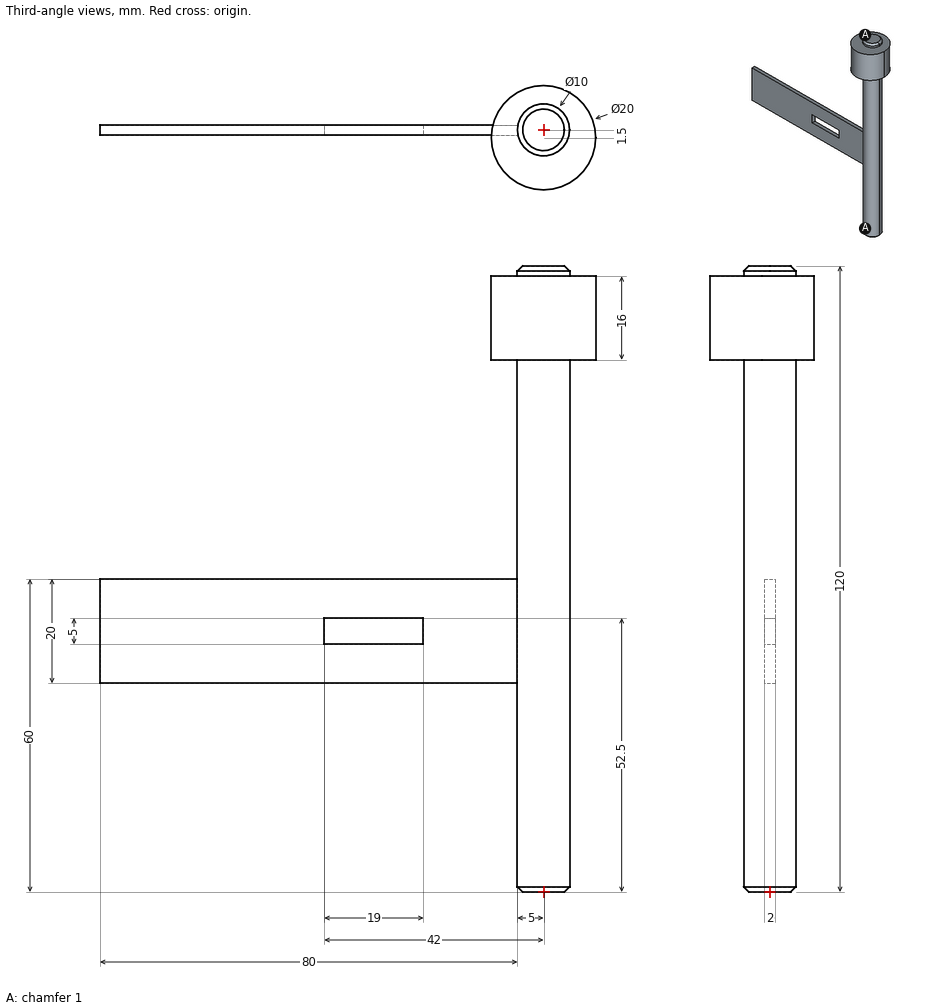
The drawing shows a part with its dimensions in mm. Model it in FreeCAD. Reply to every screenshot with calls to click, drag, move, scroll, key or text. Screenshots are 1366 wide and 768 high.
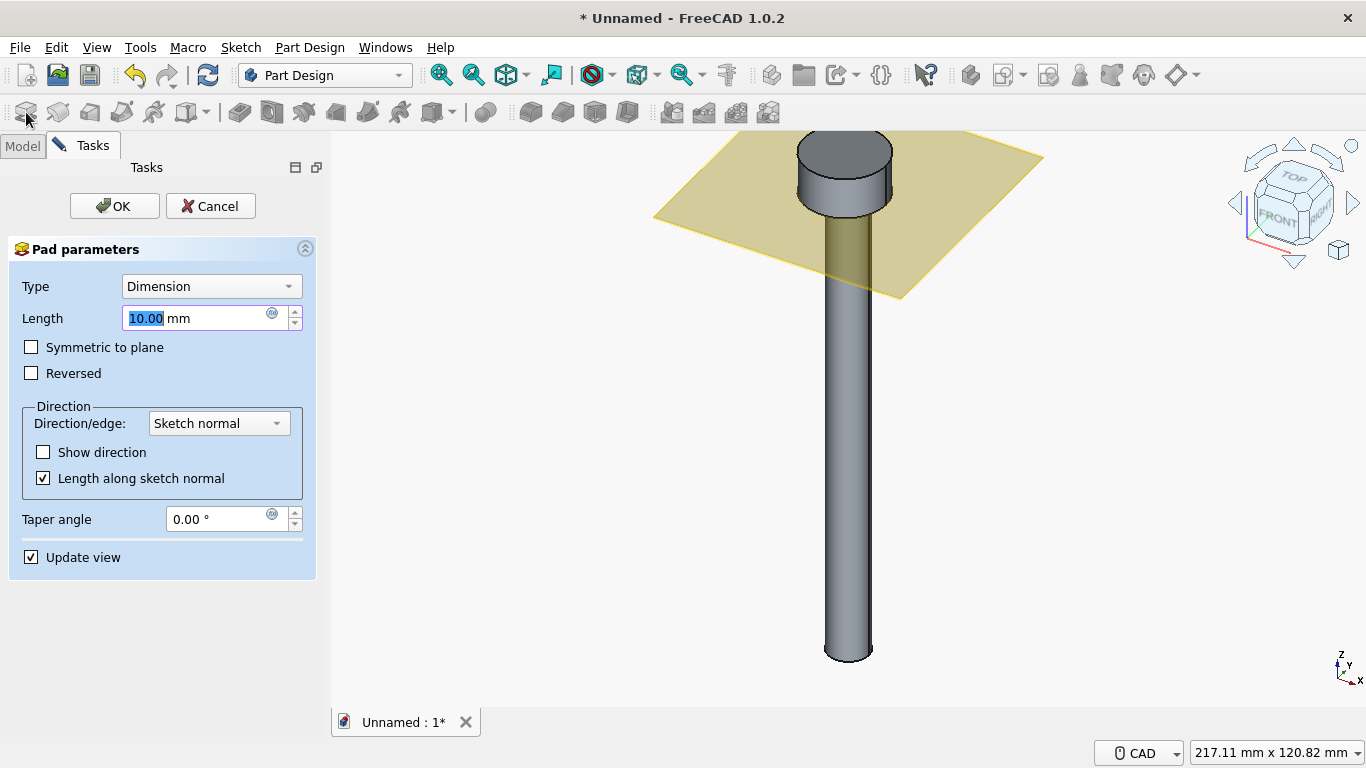
text(16)
key(Tab)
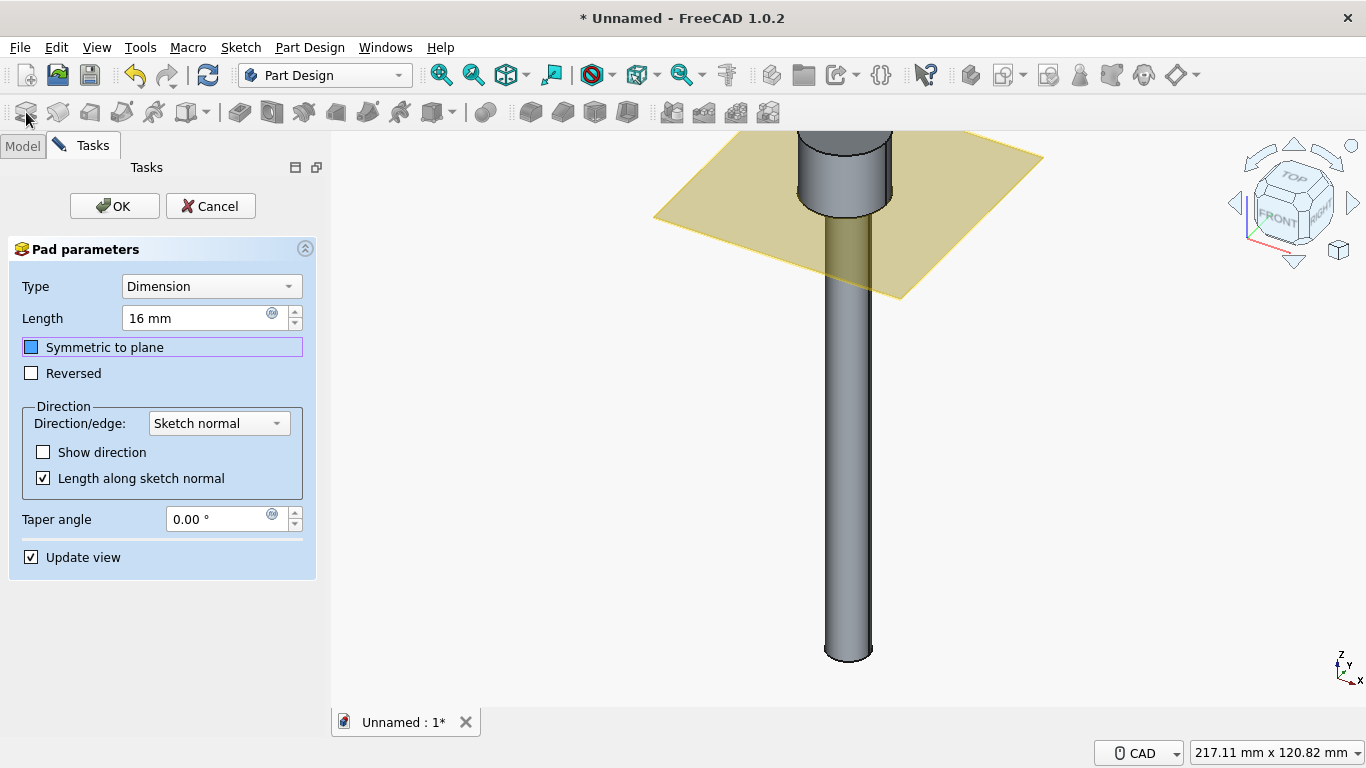
click(30, 373)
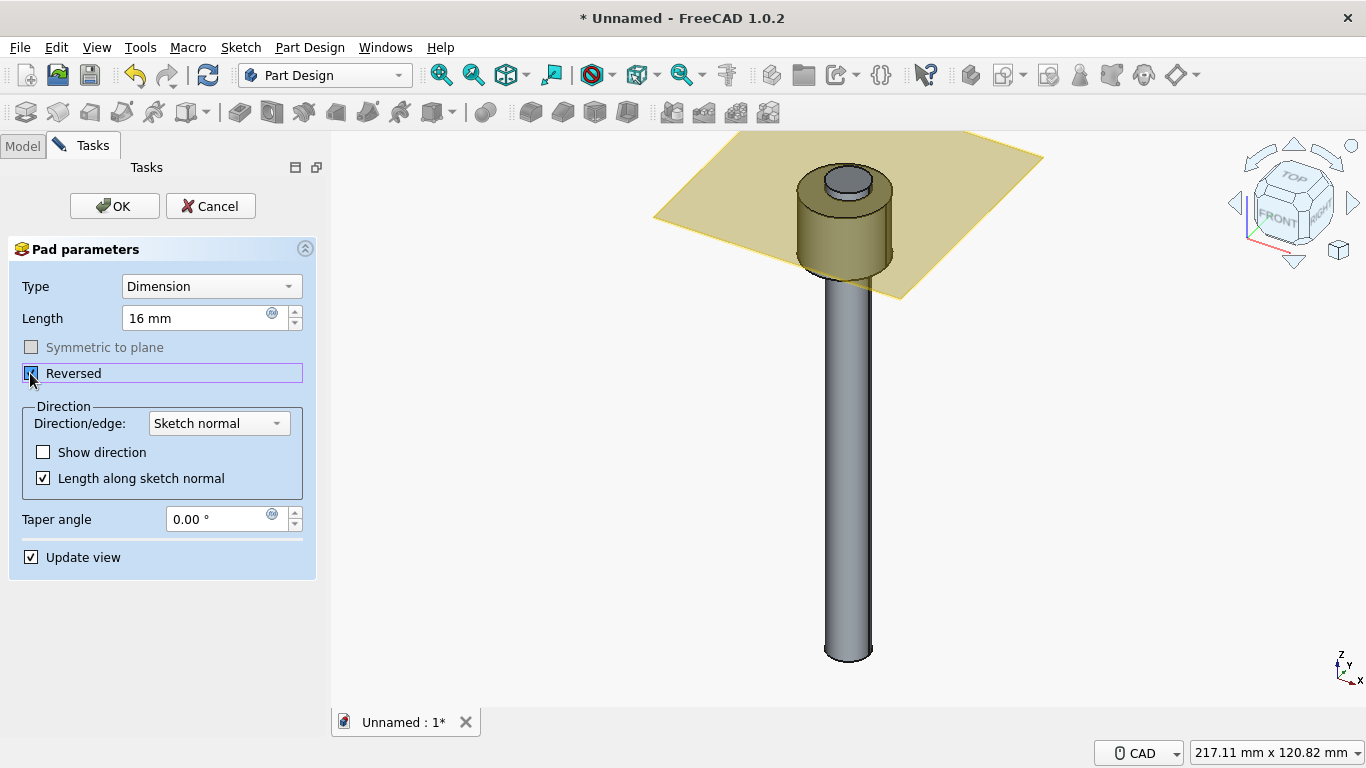
click(115, 206)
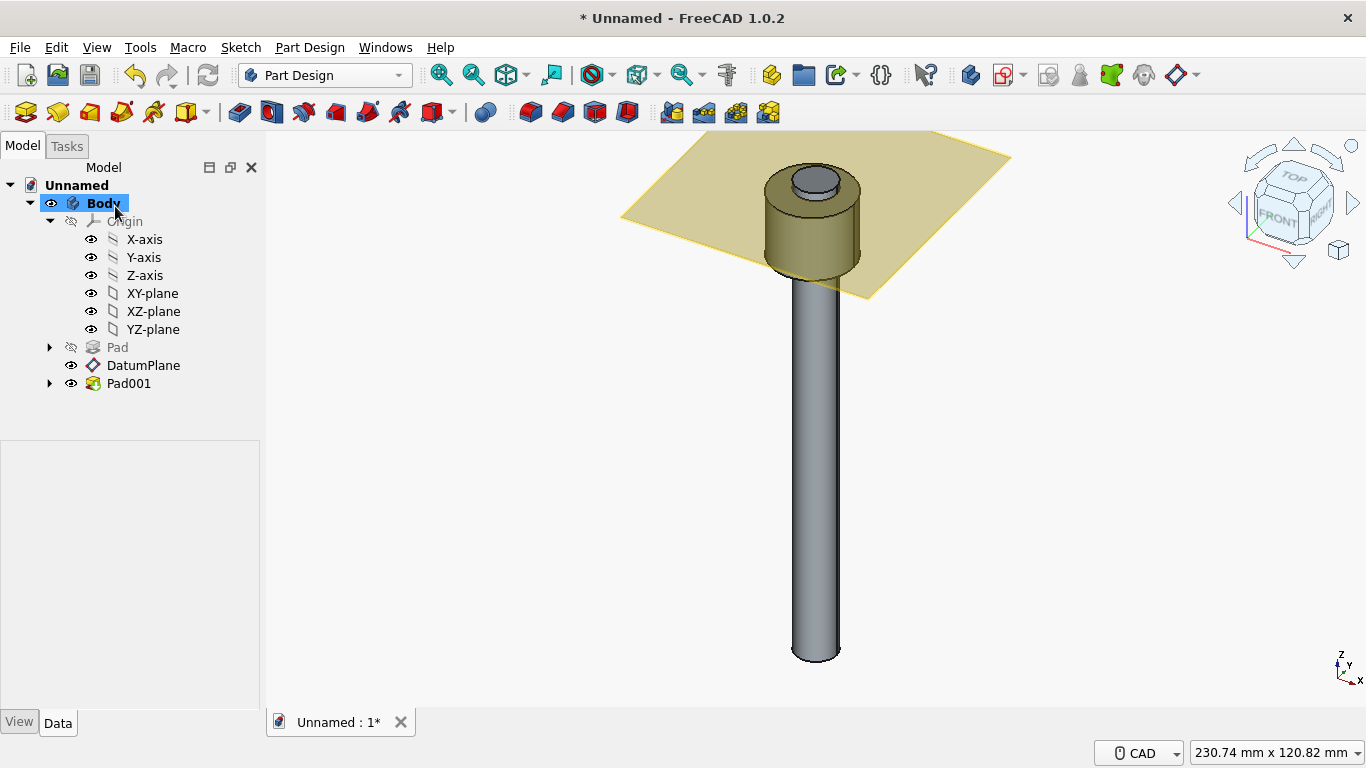
click(116, 365)
key(space)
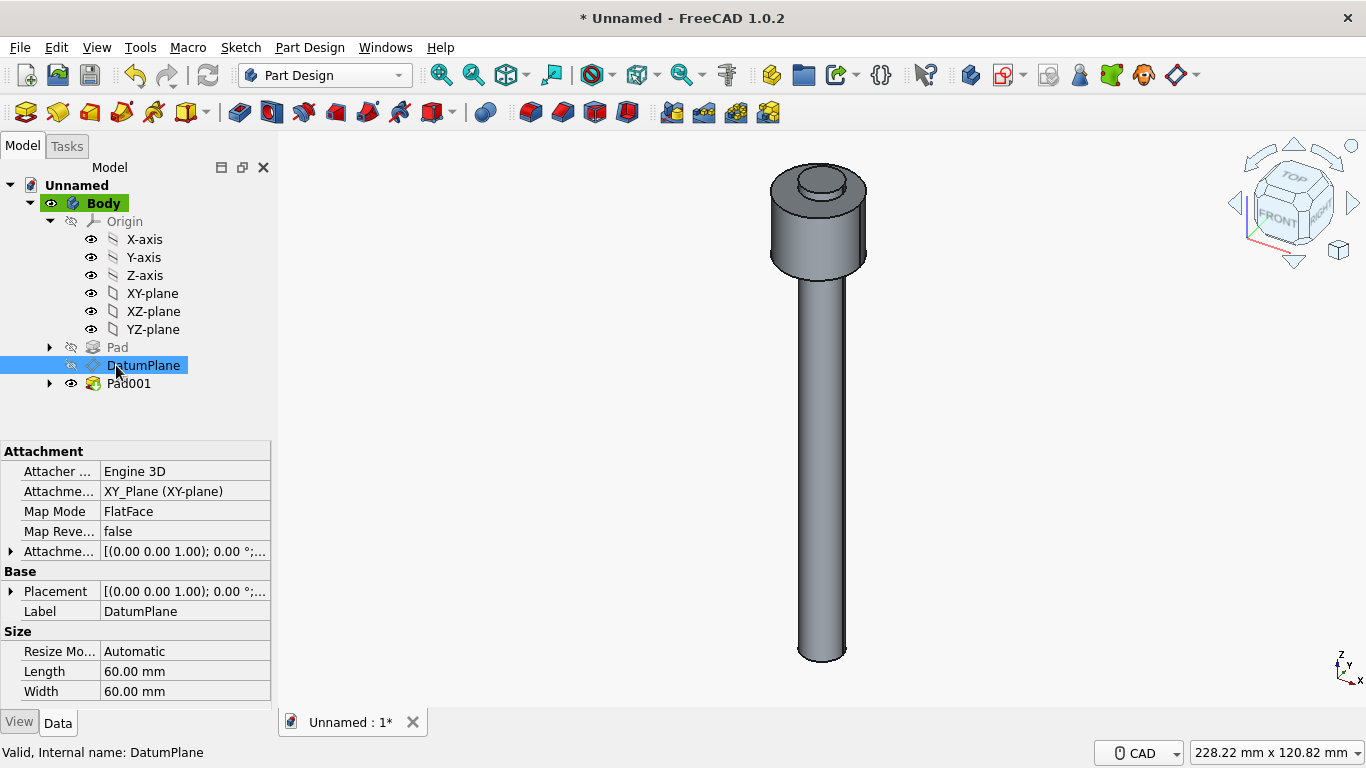
click(804, 656)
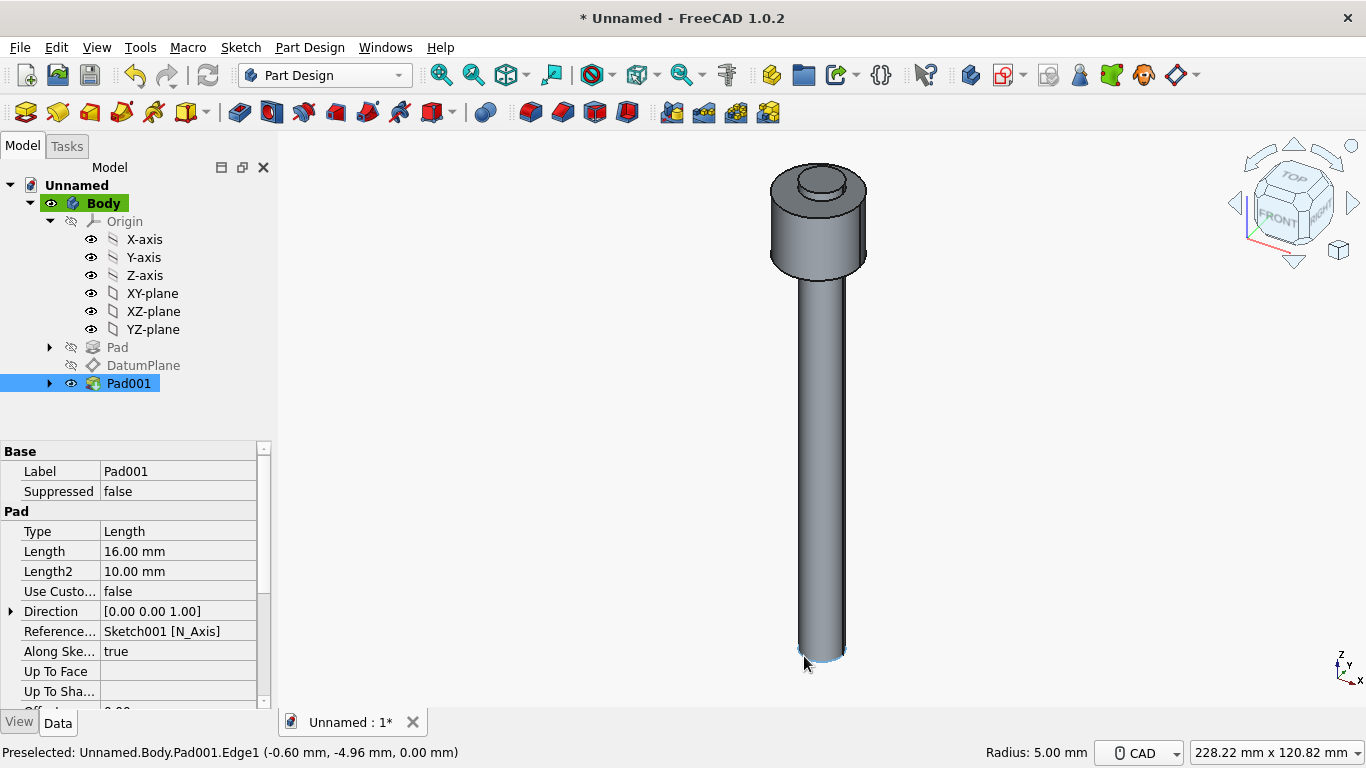
click(812, 166, ctrl)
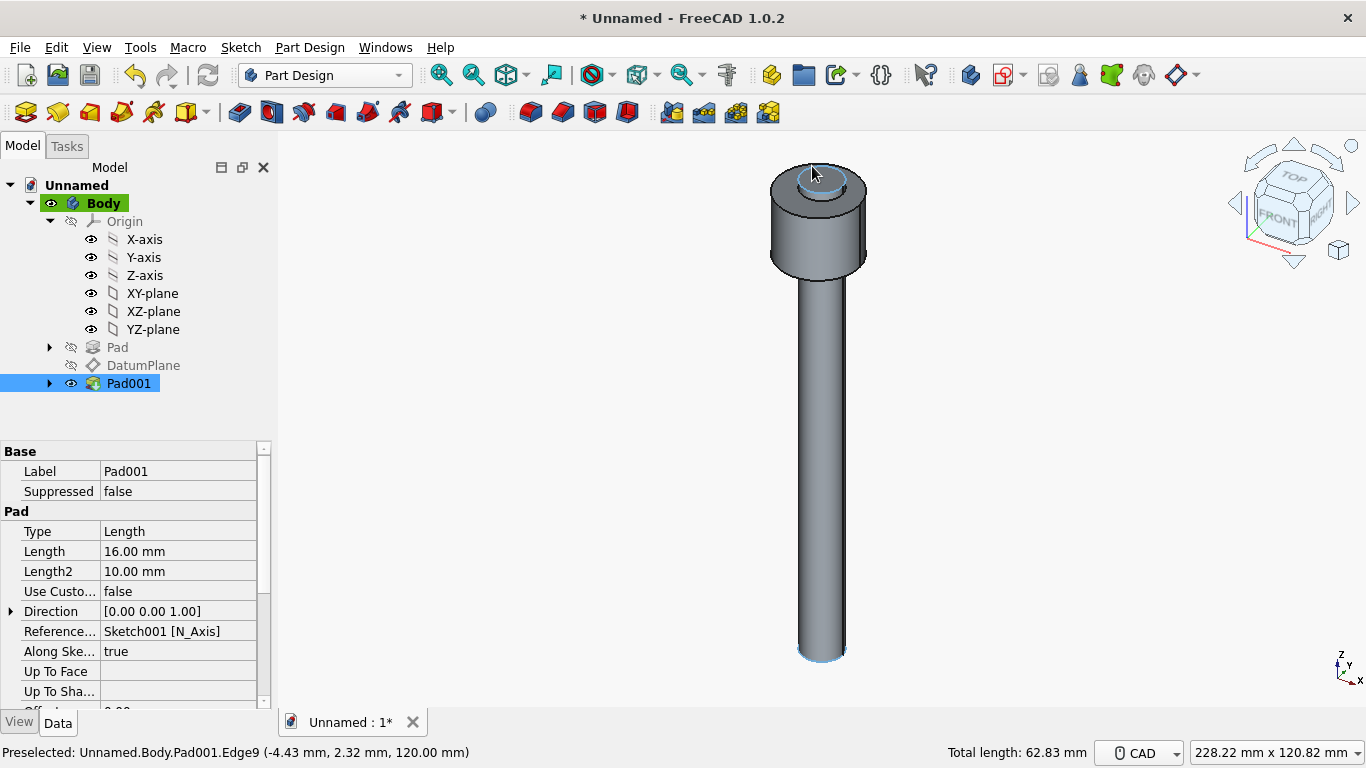
click(564, 112)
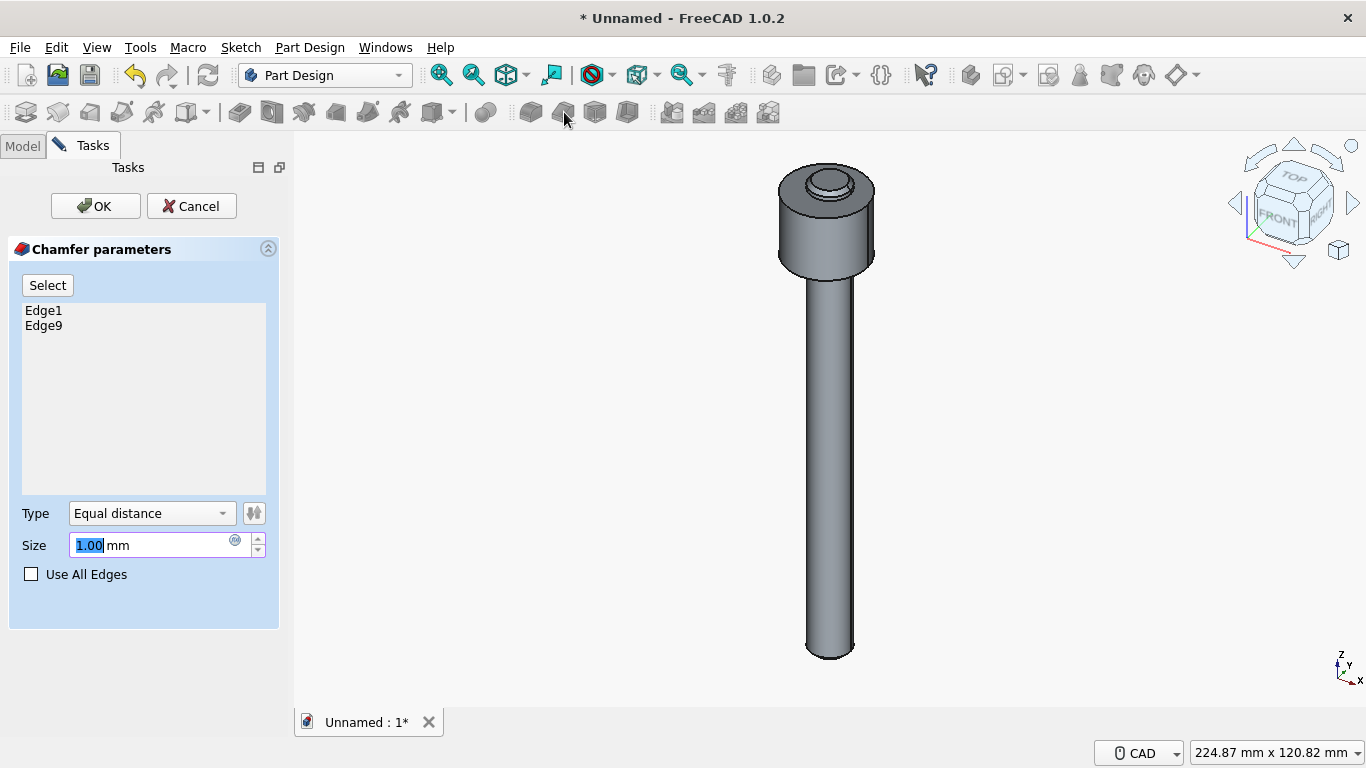
text(1)
key(Tab)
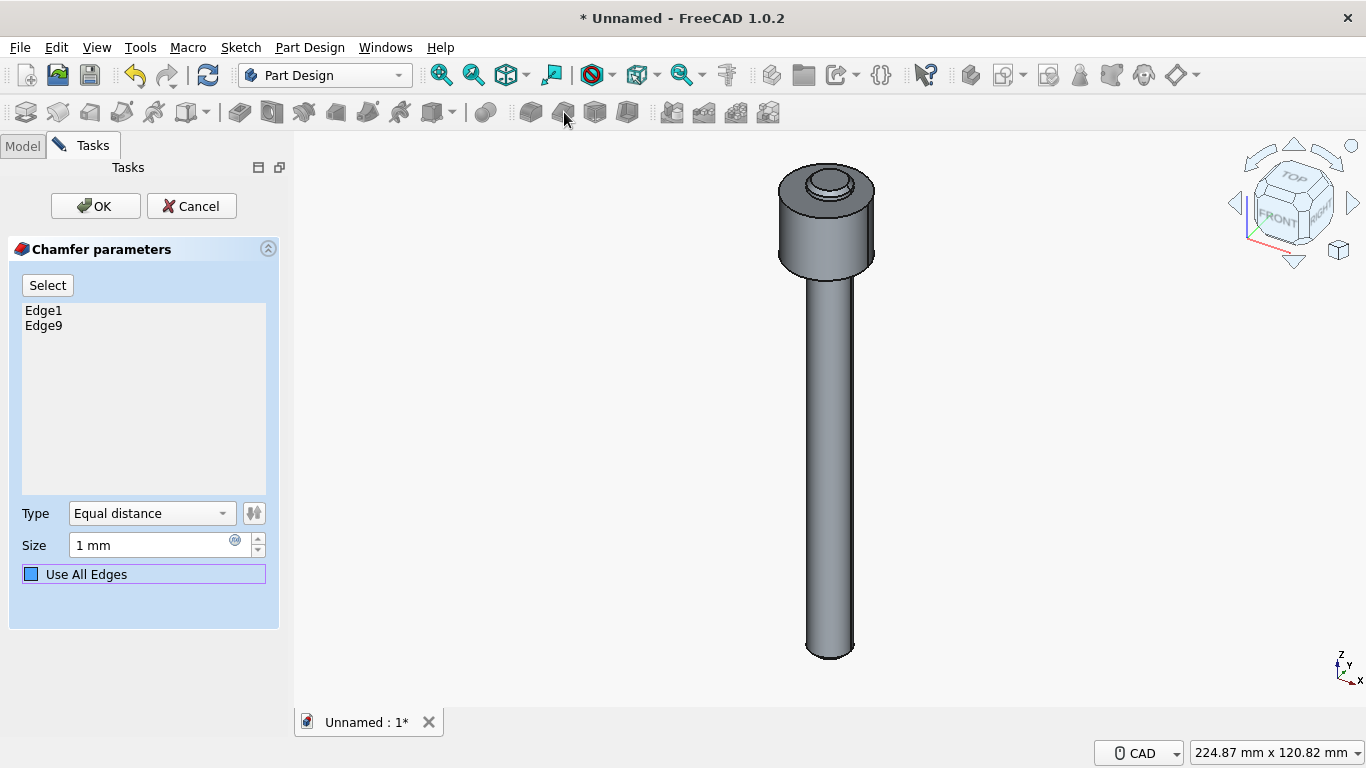
click(96, 206)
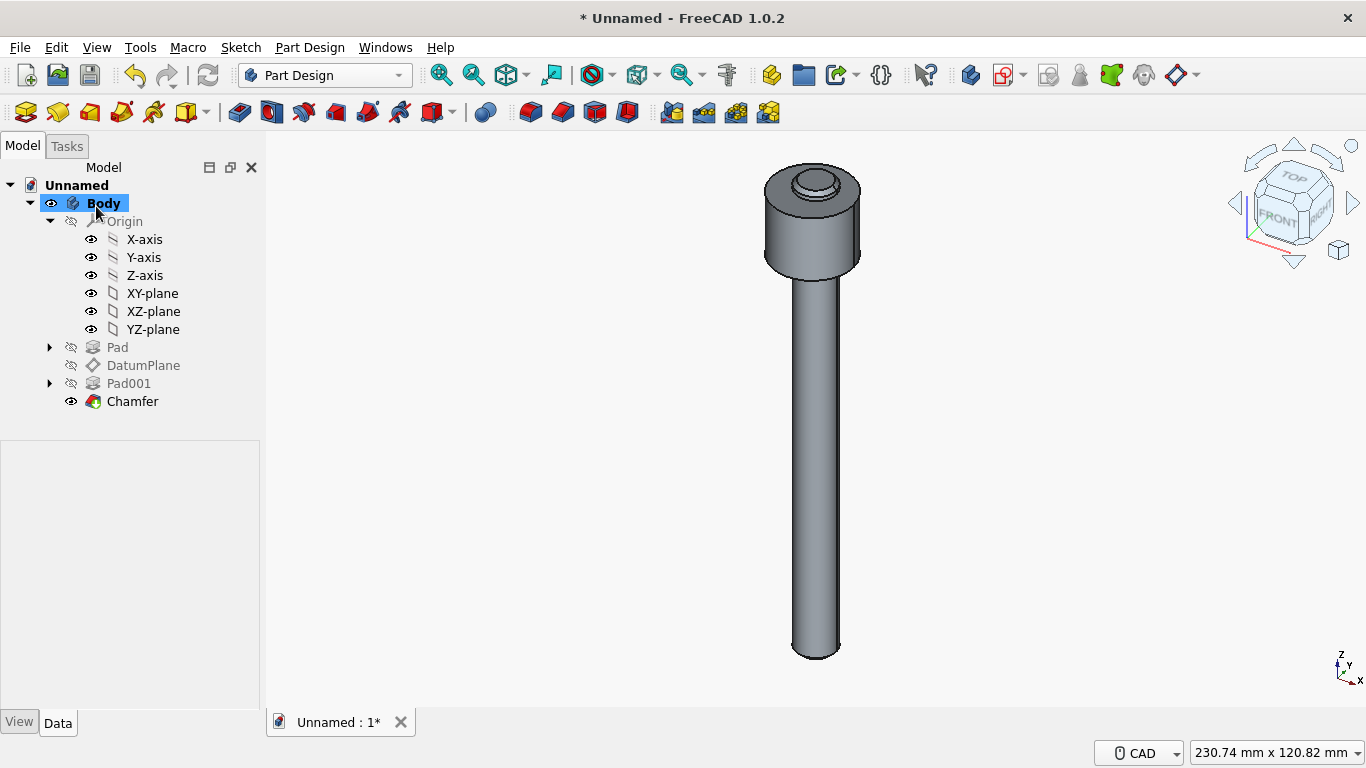
click(972, 76)